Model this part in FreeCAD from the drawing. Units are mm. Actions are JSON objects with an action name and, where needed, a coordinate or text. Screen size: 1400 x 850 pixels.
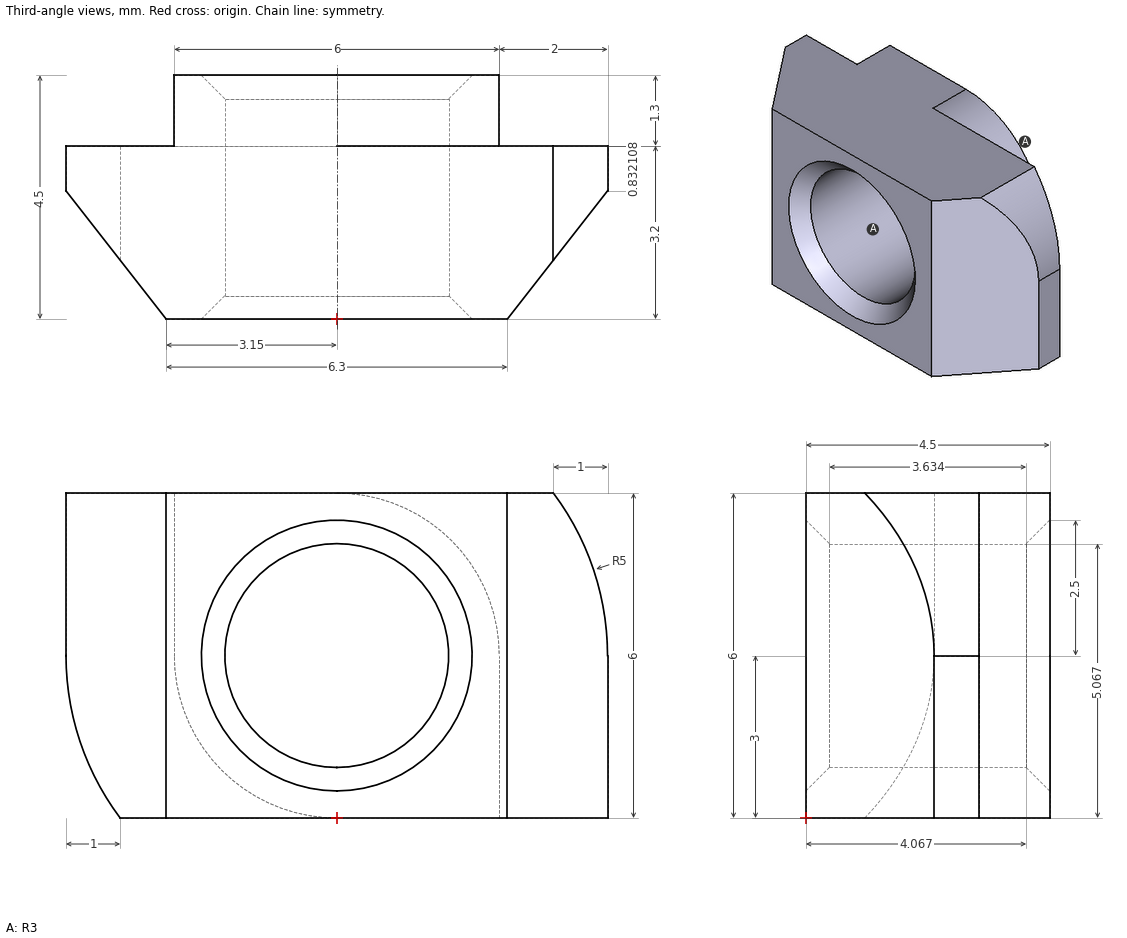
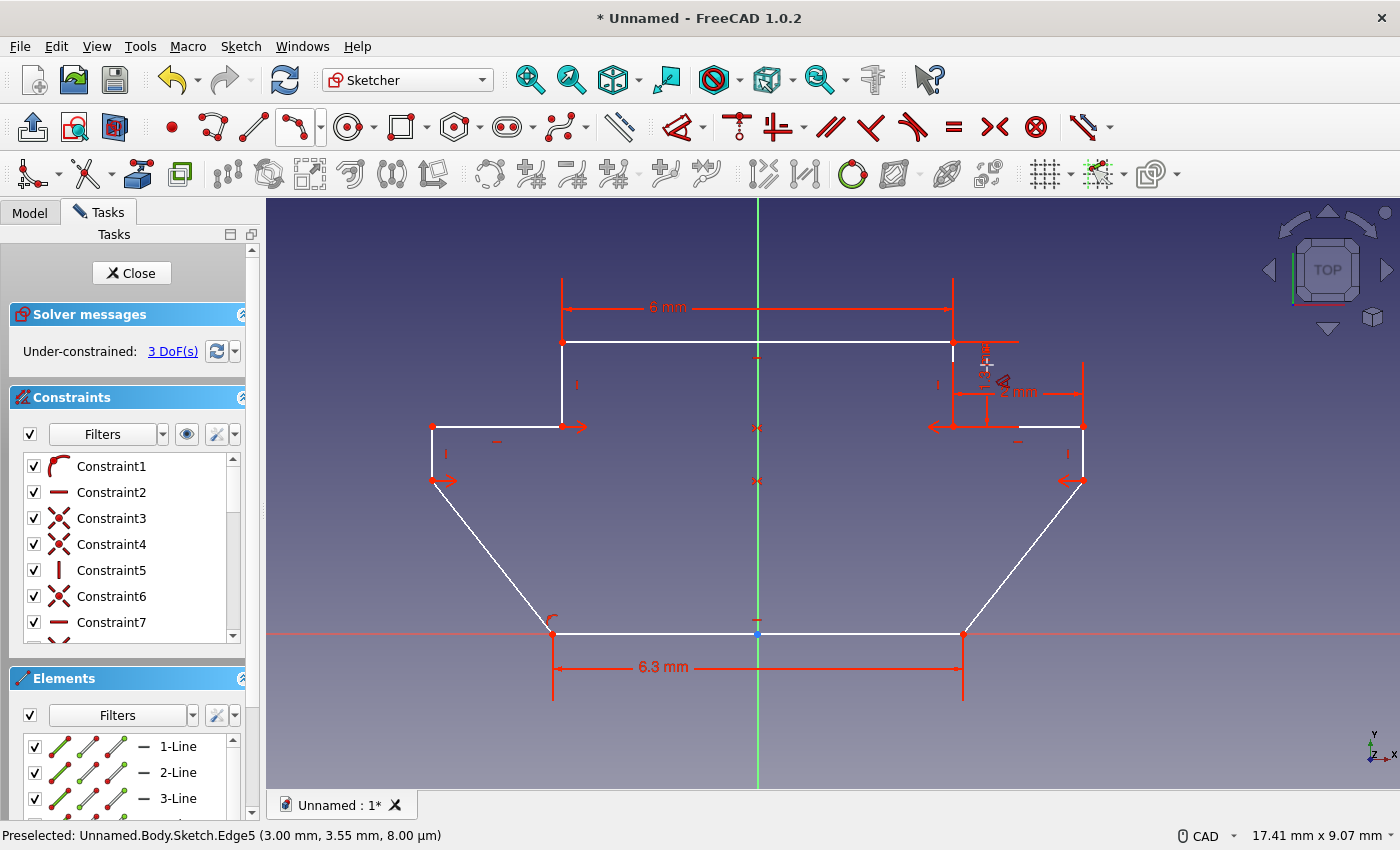
{"action": "left_click", "coordinate": [1083, 427]}
{"action": "left_click", "coordinate": [1117, 531]}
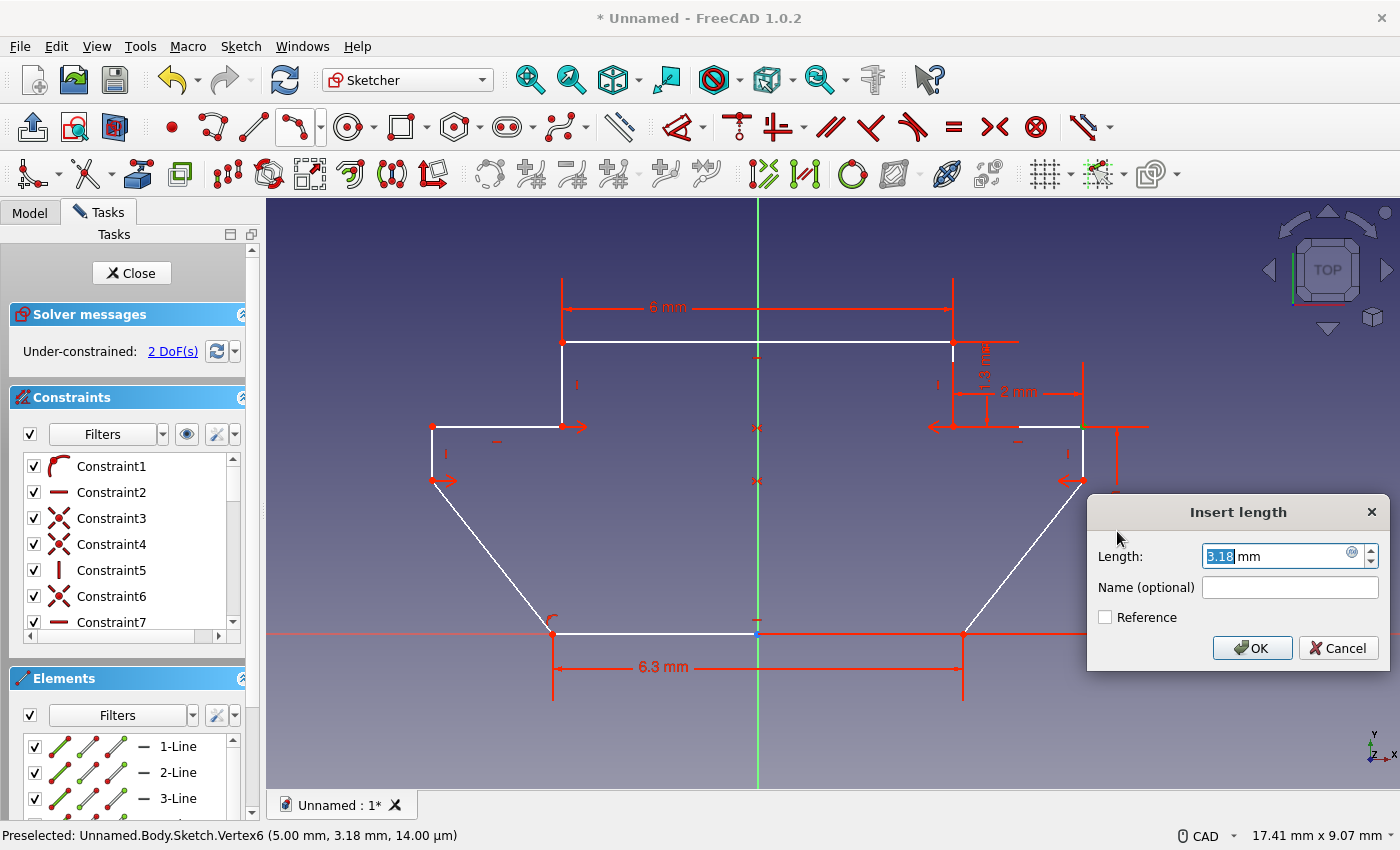
{"action": "type", "text": "3.2"}
{"action": "key", "text": "Return"}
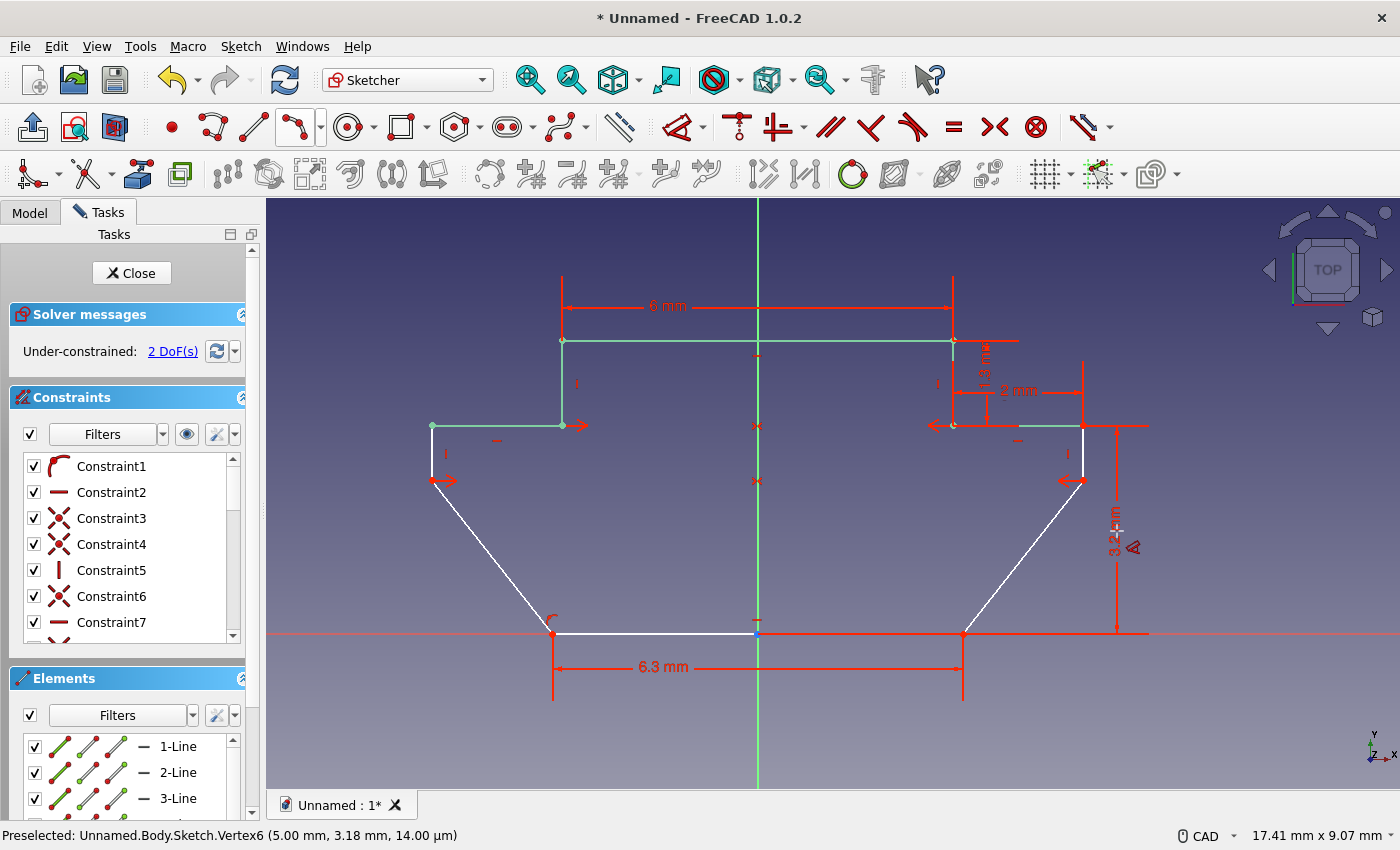
{"action": "left_click", "coordinate": [553, 634]}
{"action": "left_click", "coordinate": [583, 668]}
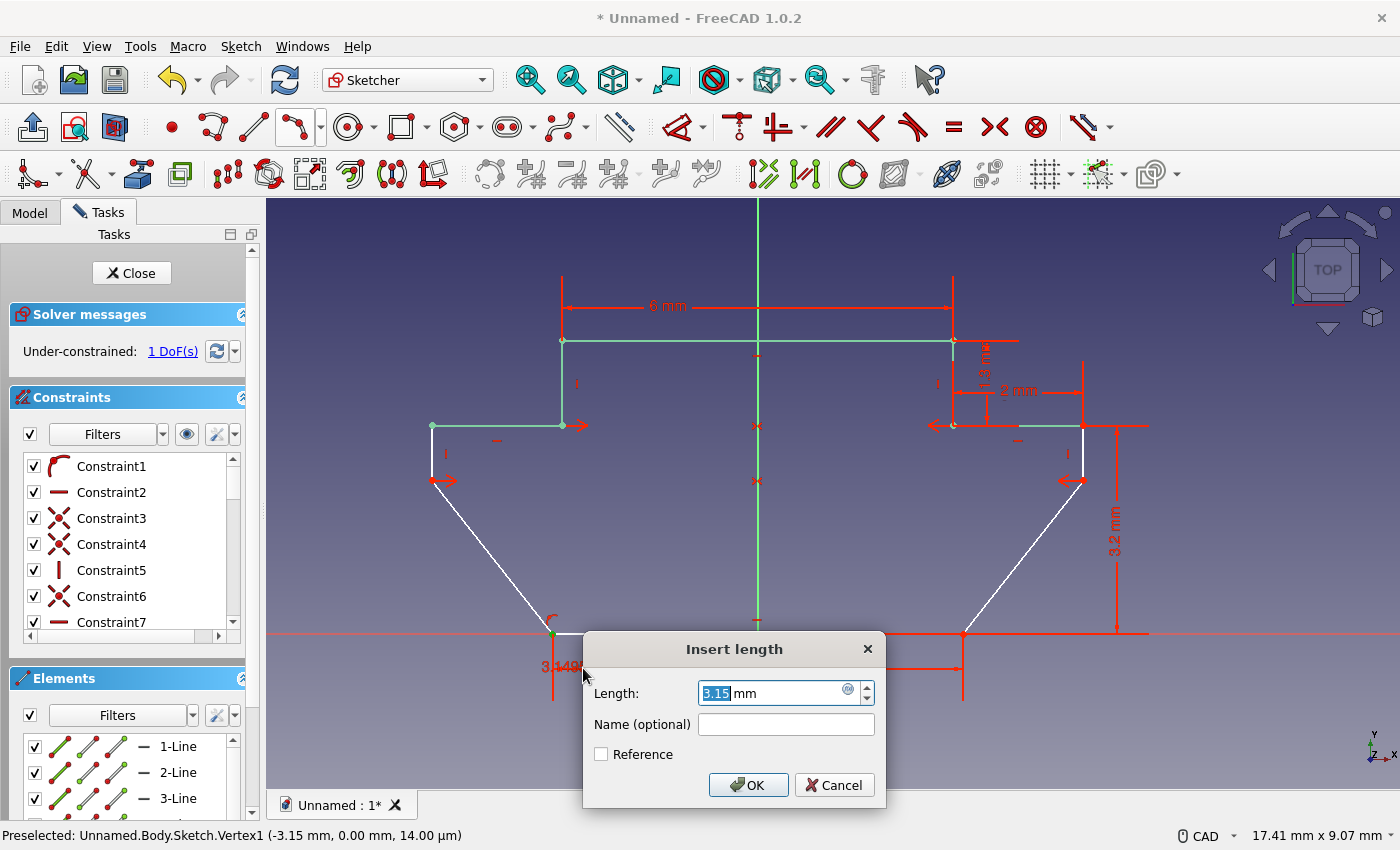
{"action": "type", "text": "3.15"}
{"action": "key", "text": "Return"}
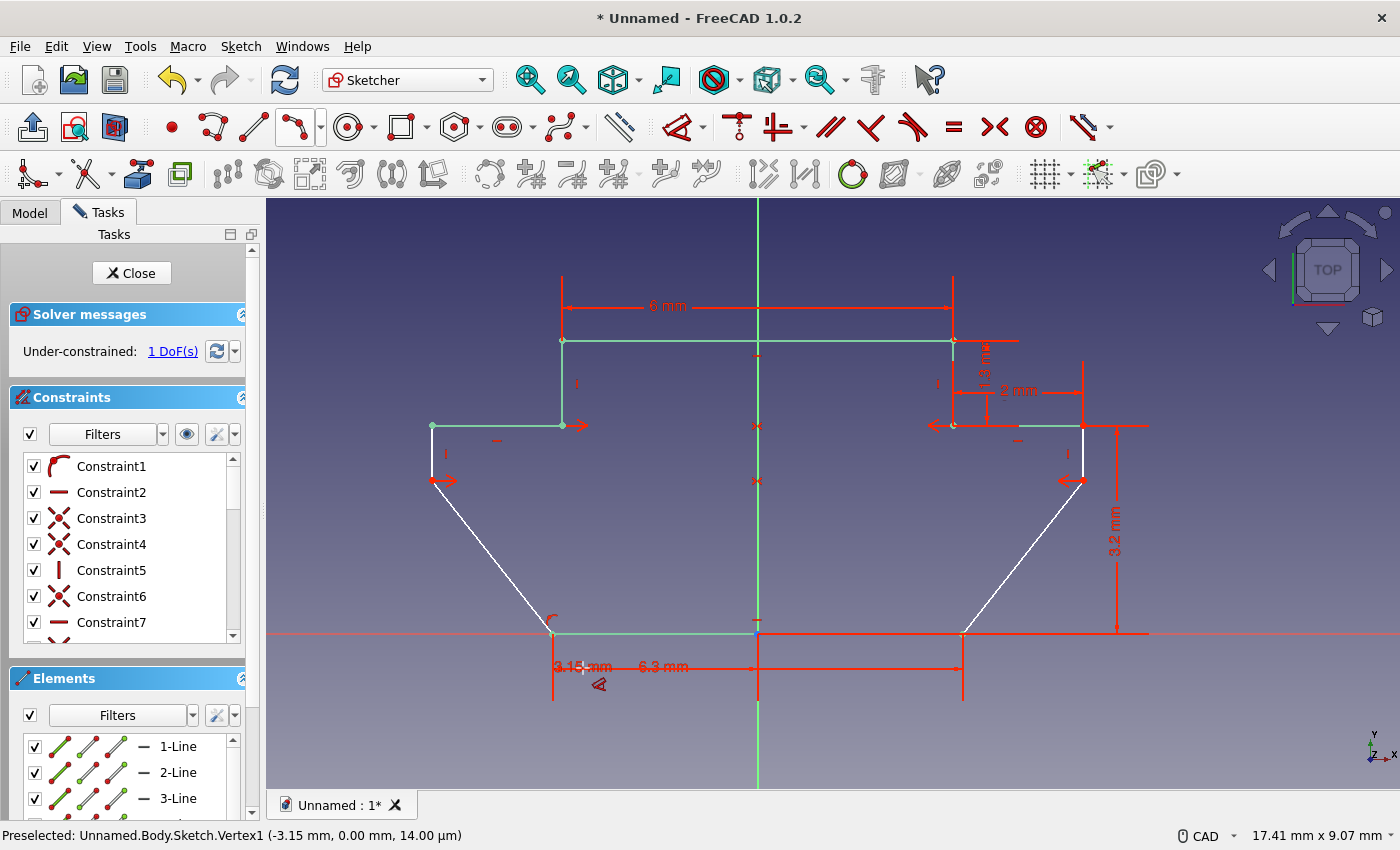
{"action": "left_click", "coordinate": [1083, 464]}
{"action": "left_click", "coordinate": [1117, 453]}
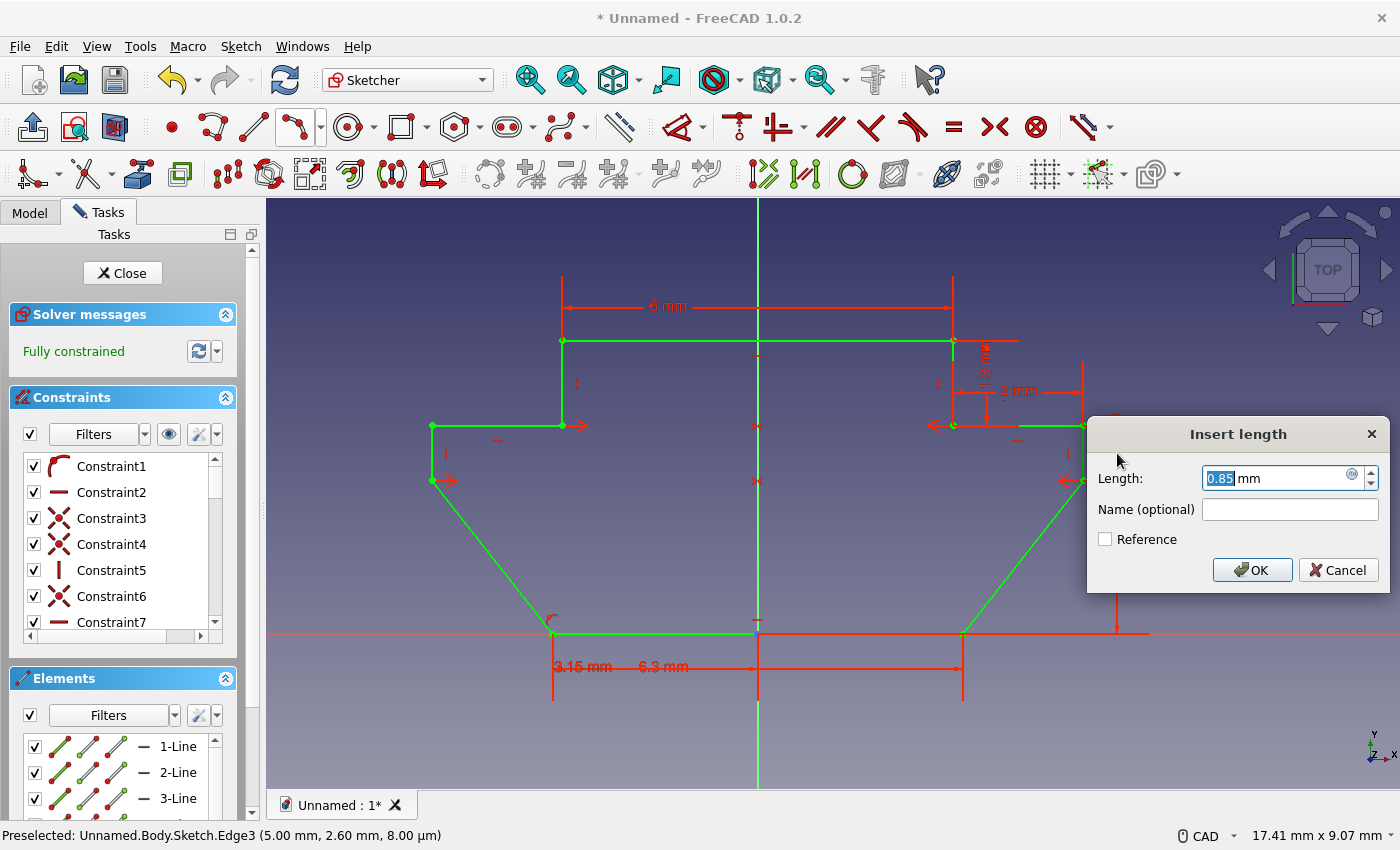
{"action": "type", "text": "0.832108"}
{"action": "key", "text": "Return"}
{"action": "key", "text": "Escape"}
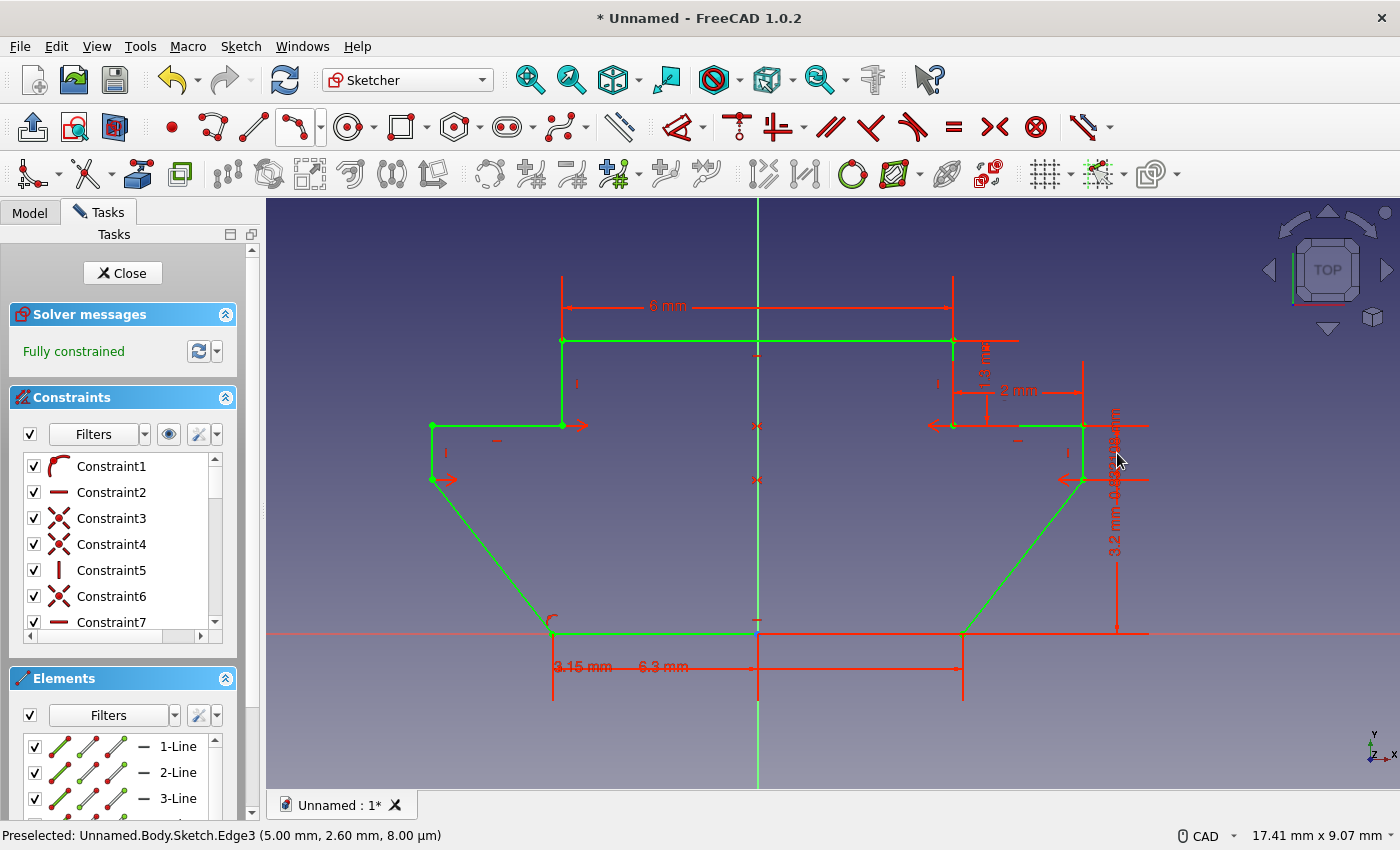
{"action": "left_click", "coordinate": [123, 273]}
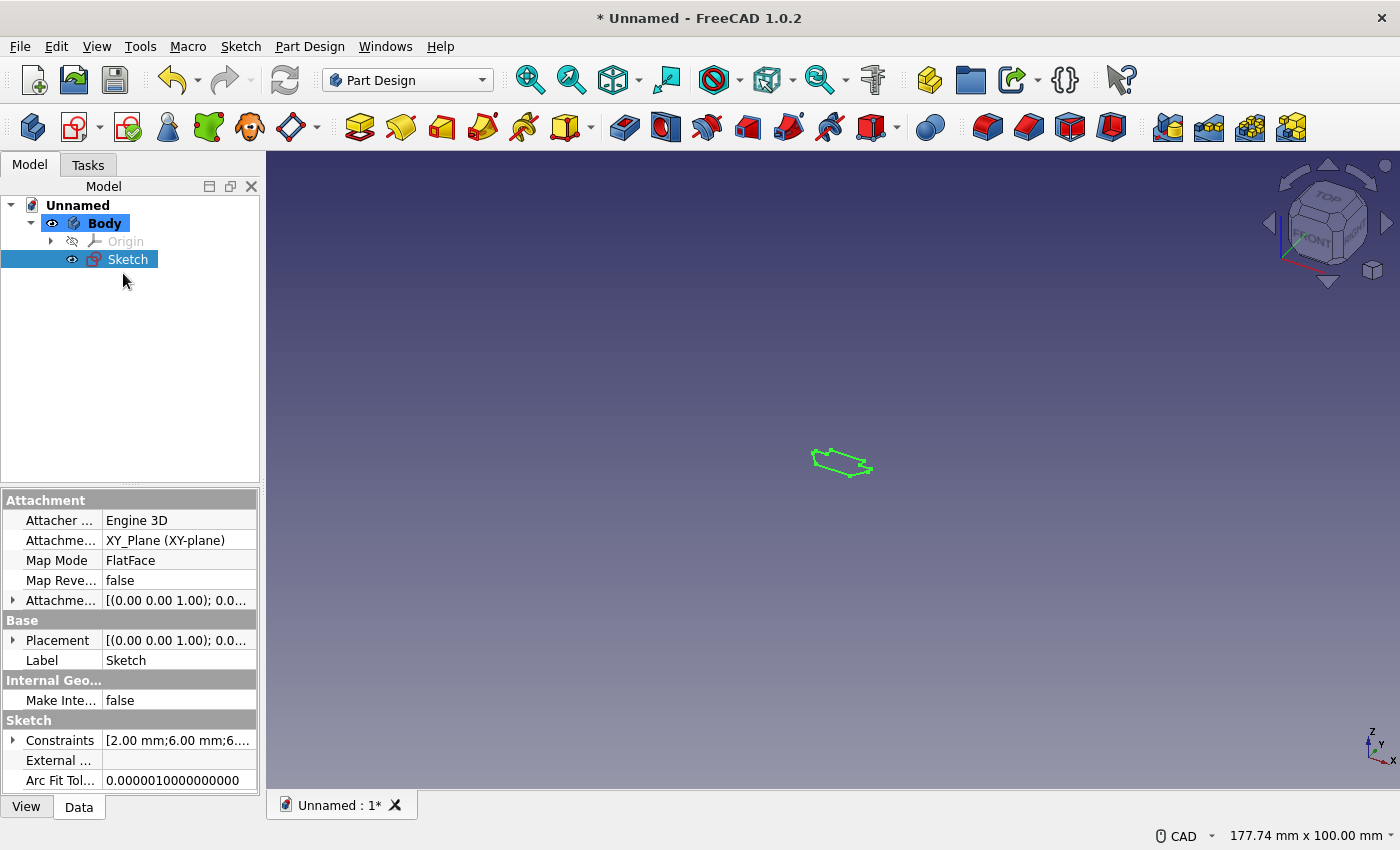
{"action": "left_click", "coordinate": [360, 128]}